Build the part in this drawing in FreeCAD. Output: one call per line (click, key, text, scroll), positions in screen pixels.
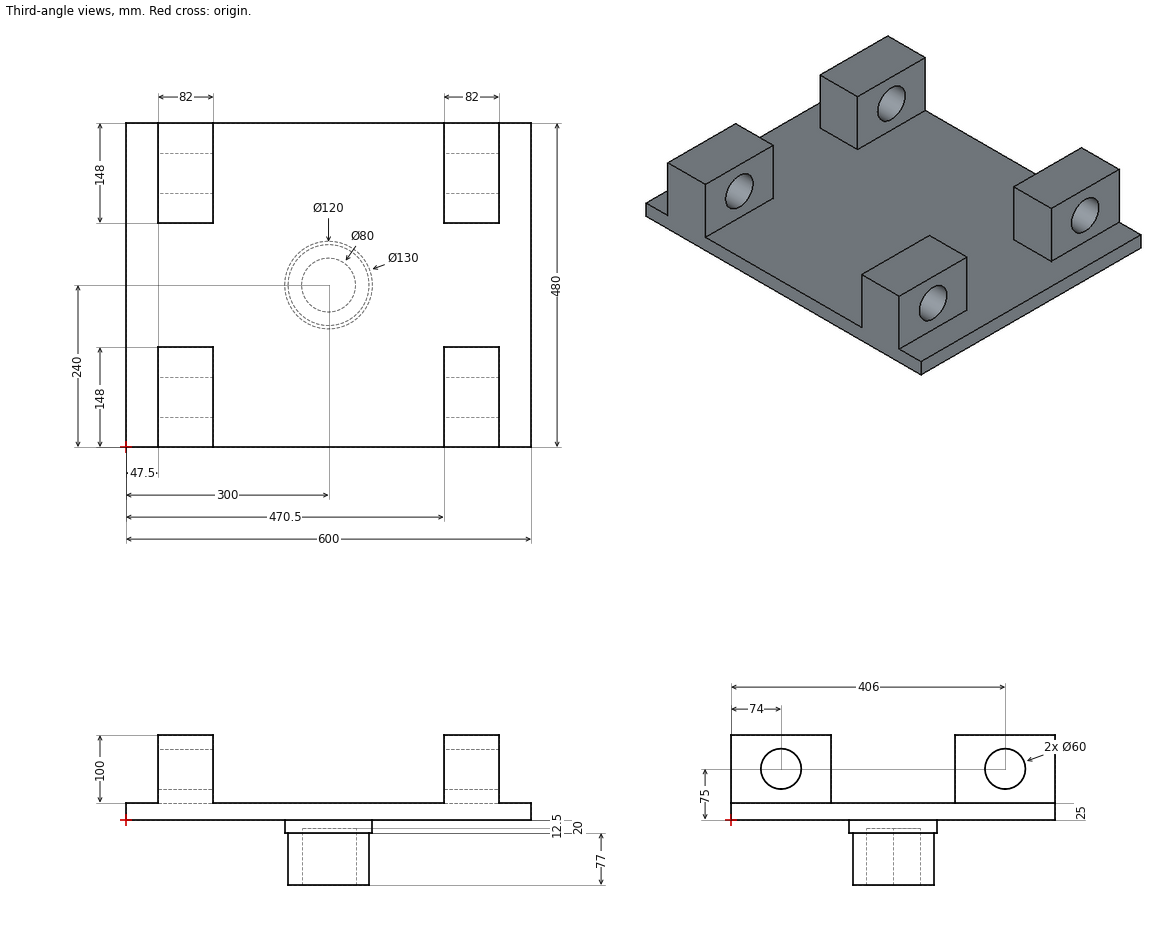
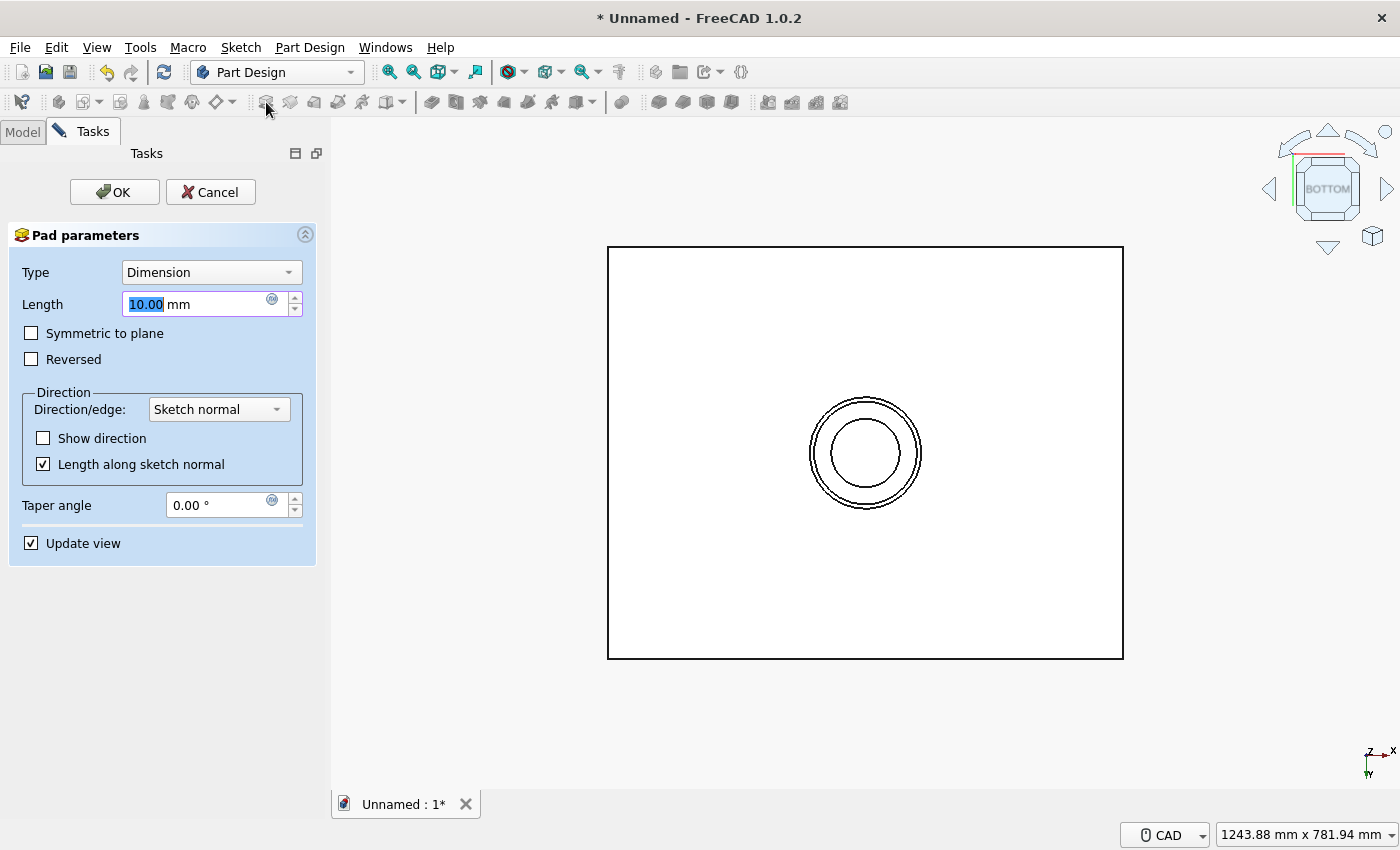
text(77)
key(Tab)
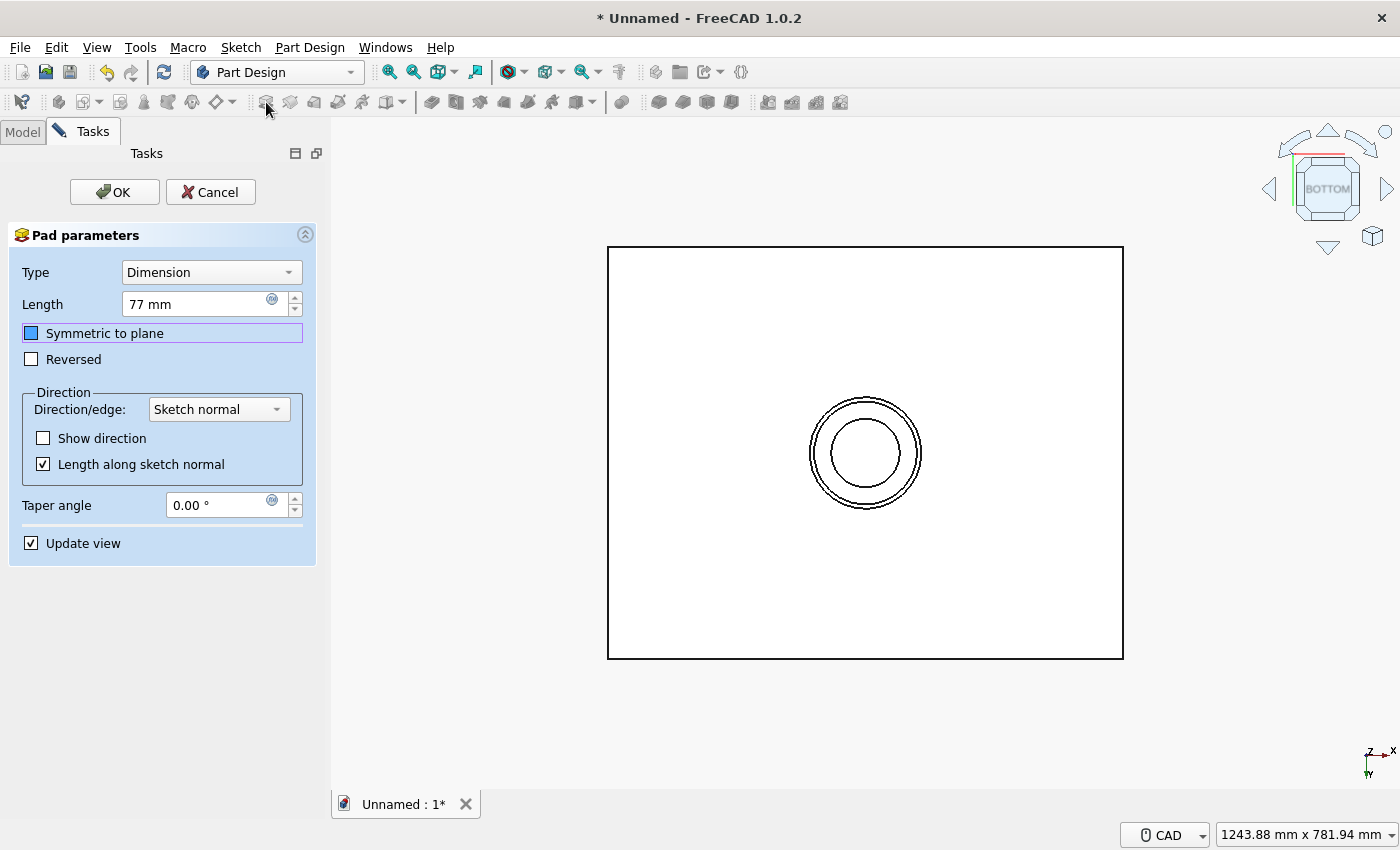
click(115, 192)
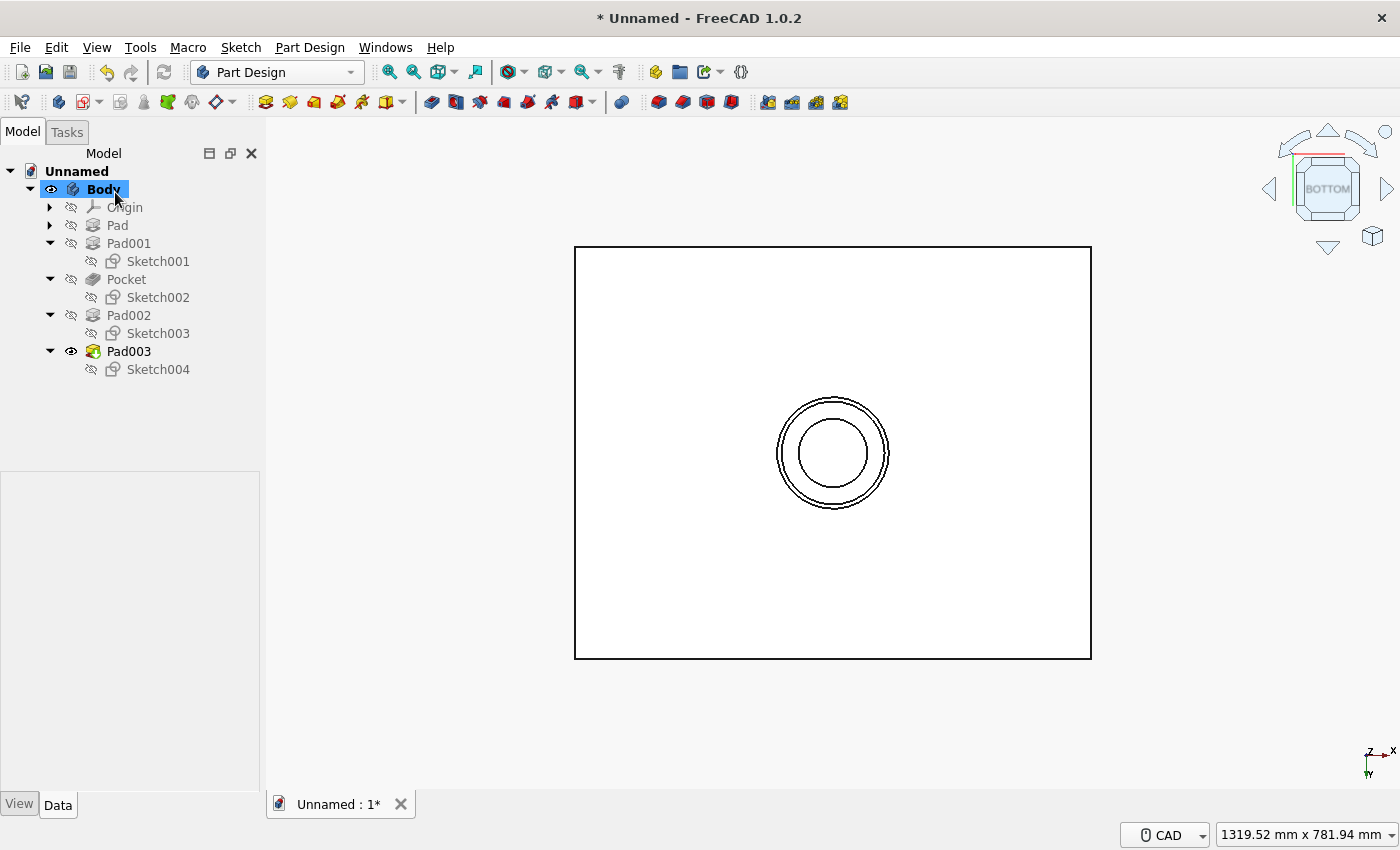
click(980, 393)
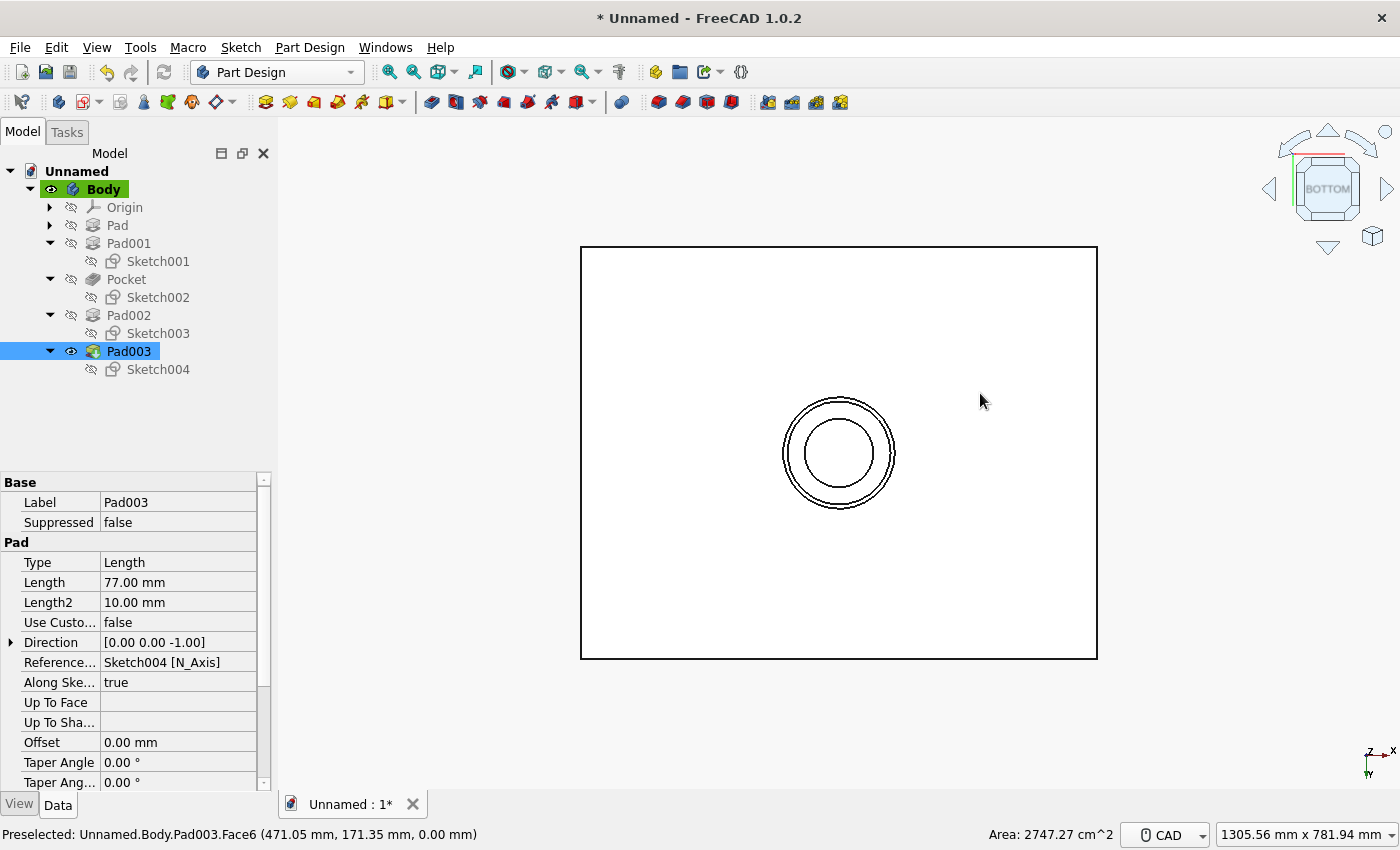
click(84, 102)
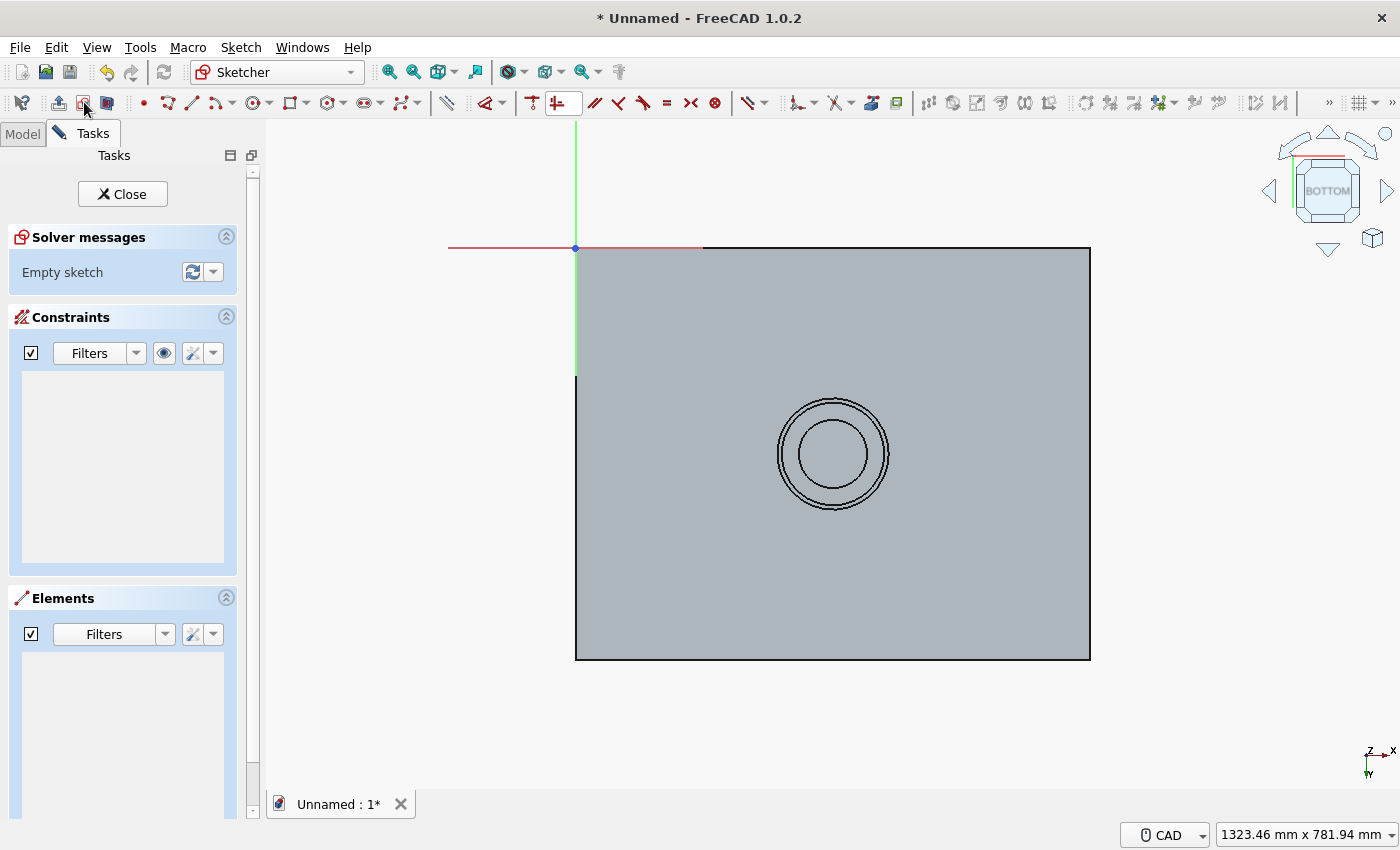
click(108, 104)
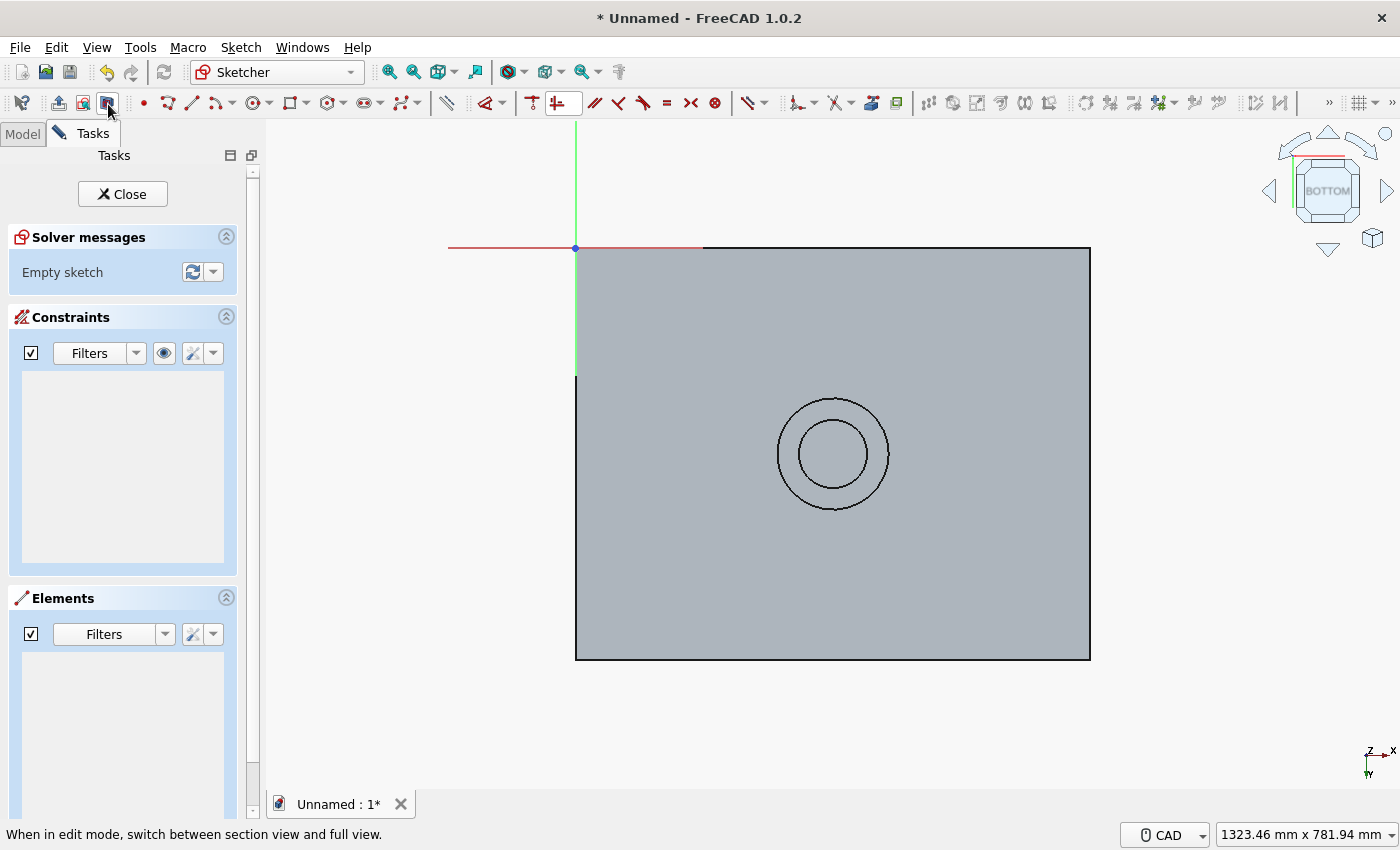
scroll(847, 454, up, 9)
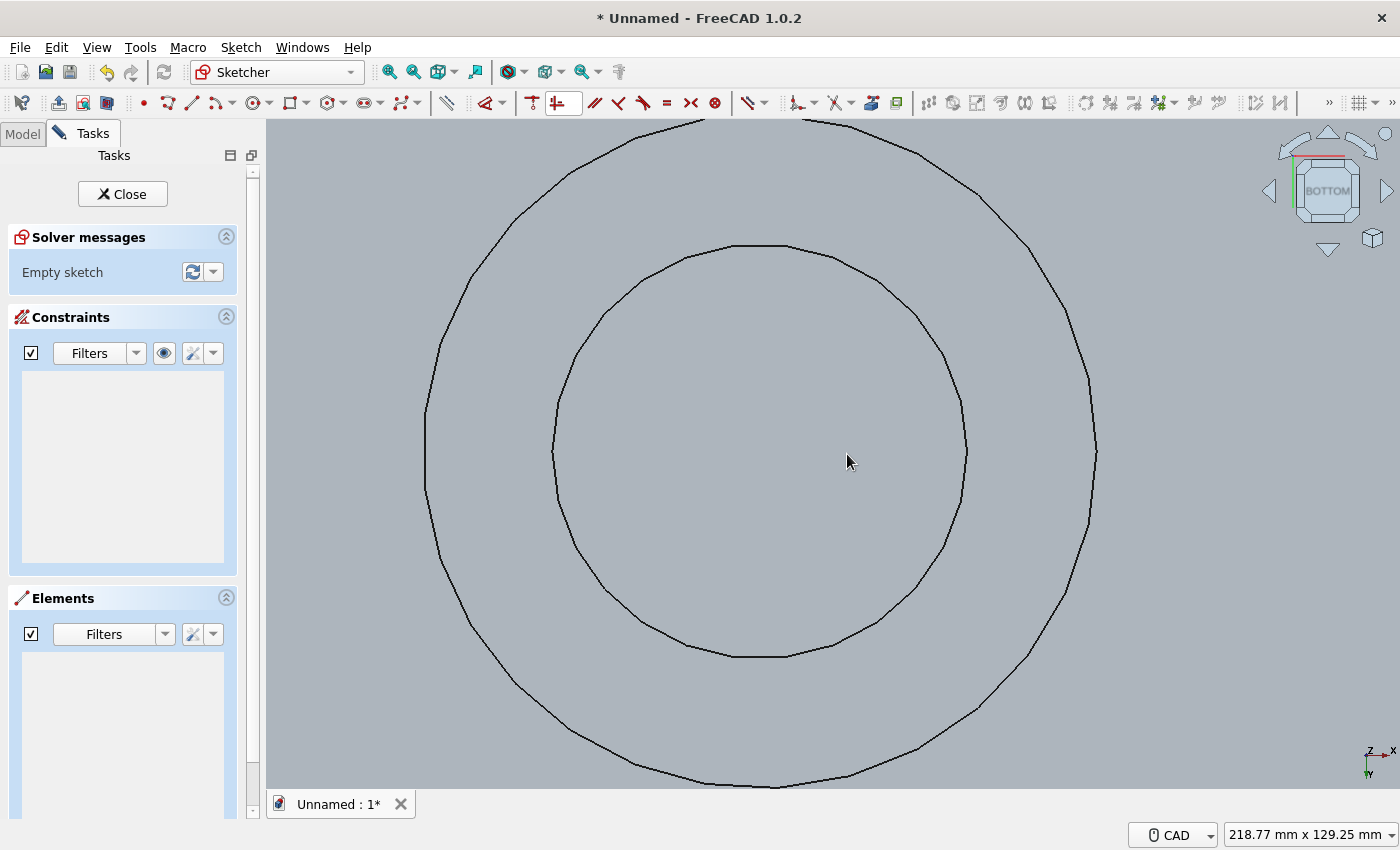
key(g)
key(c)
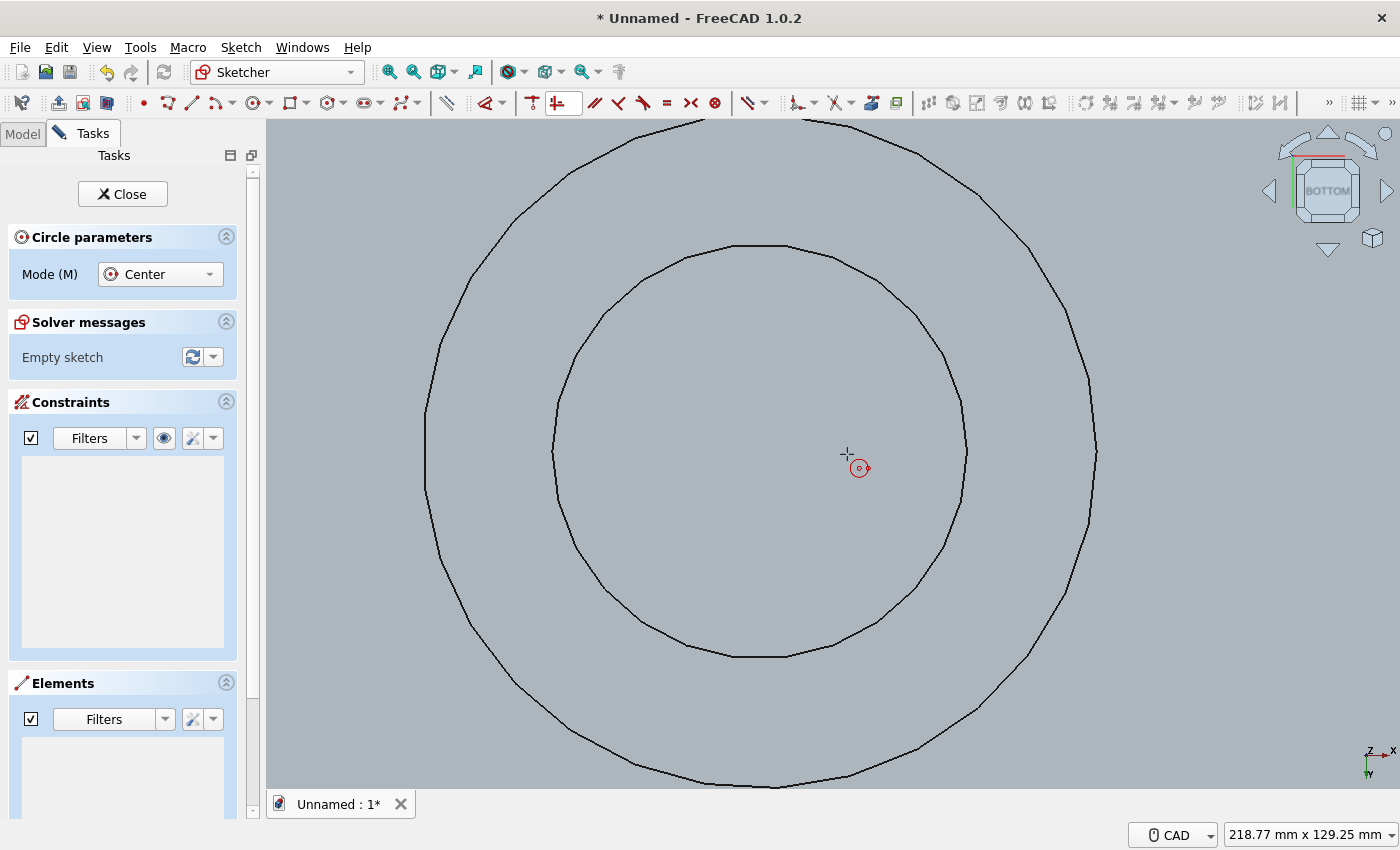
click(760, 451)
move(906, 305)